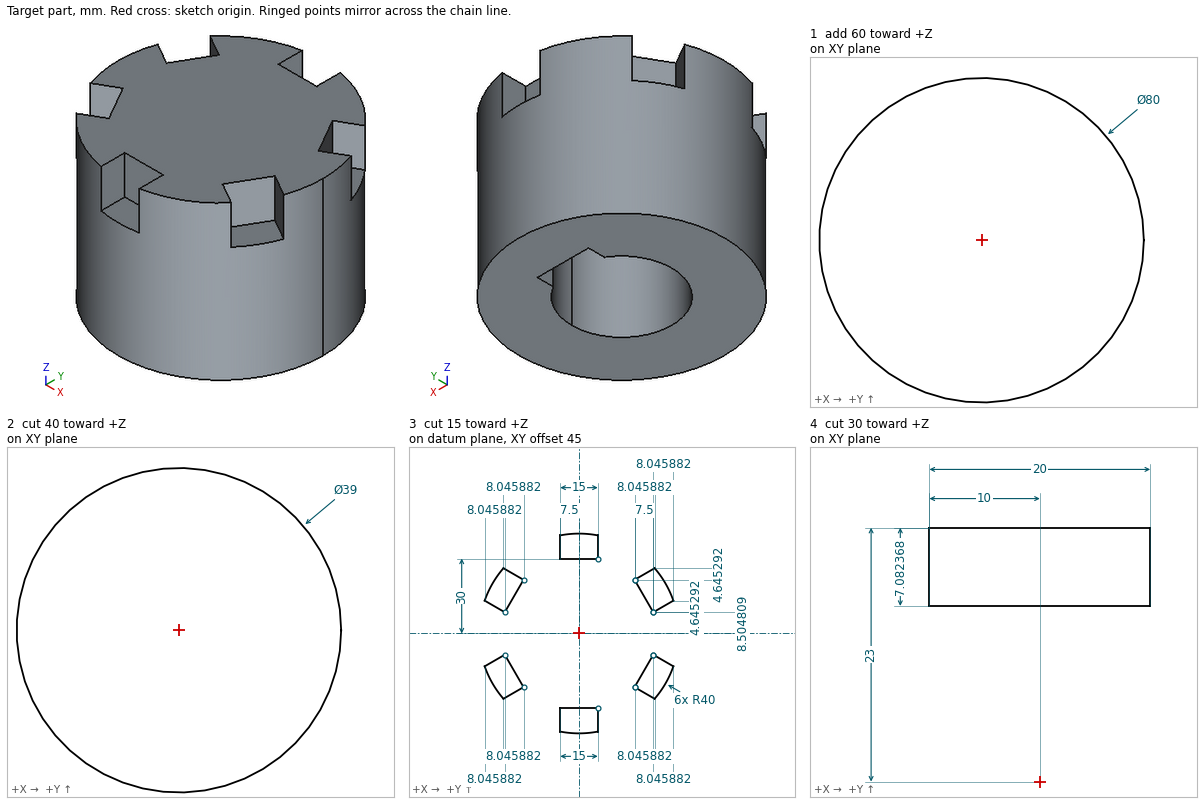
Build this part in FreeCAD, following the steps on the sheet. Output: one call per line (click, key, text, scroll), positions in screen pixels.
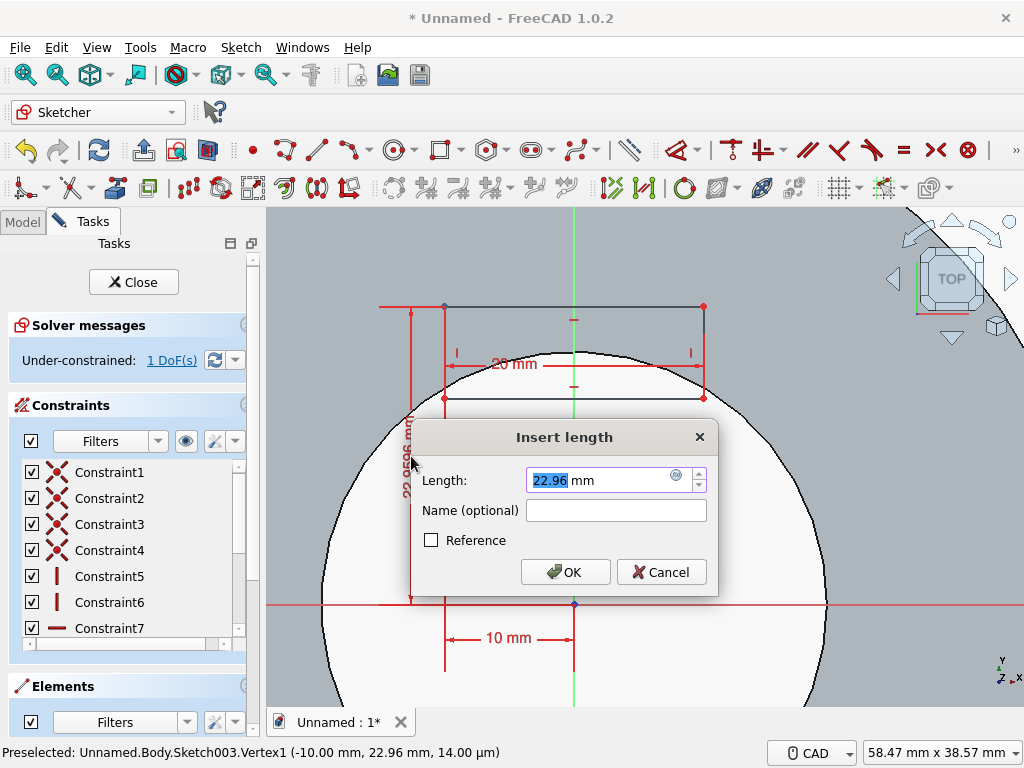
text(23)
key(Return)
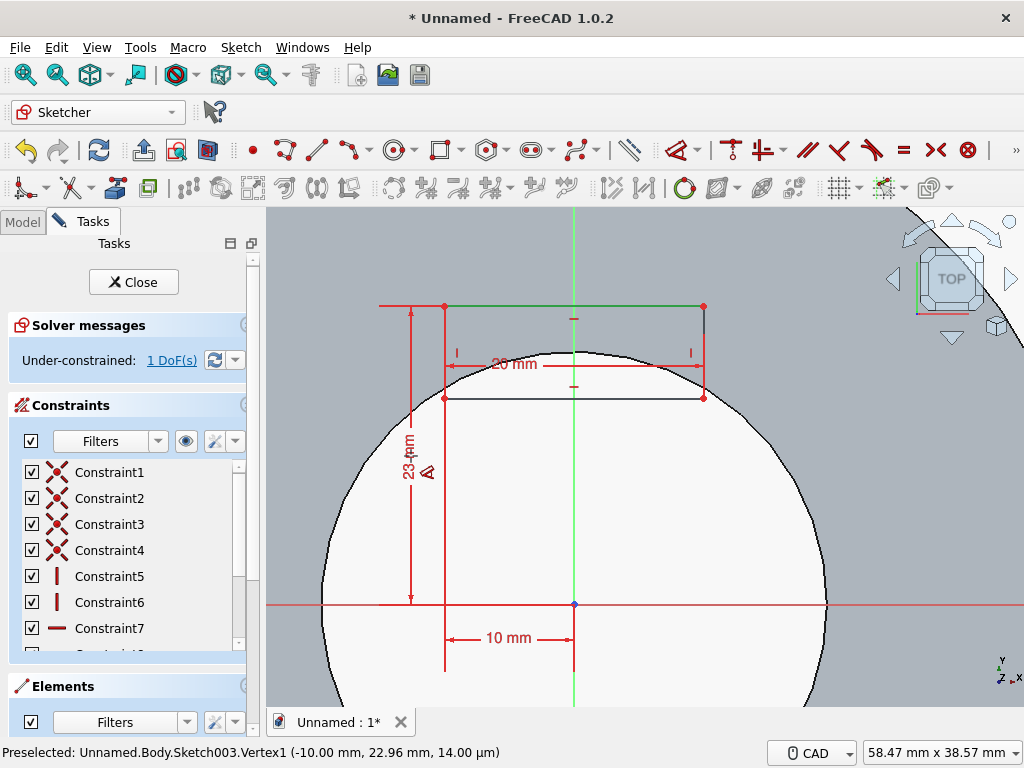
click(445, 334)
click(411, 353)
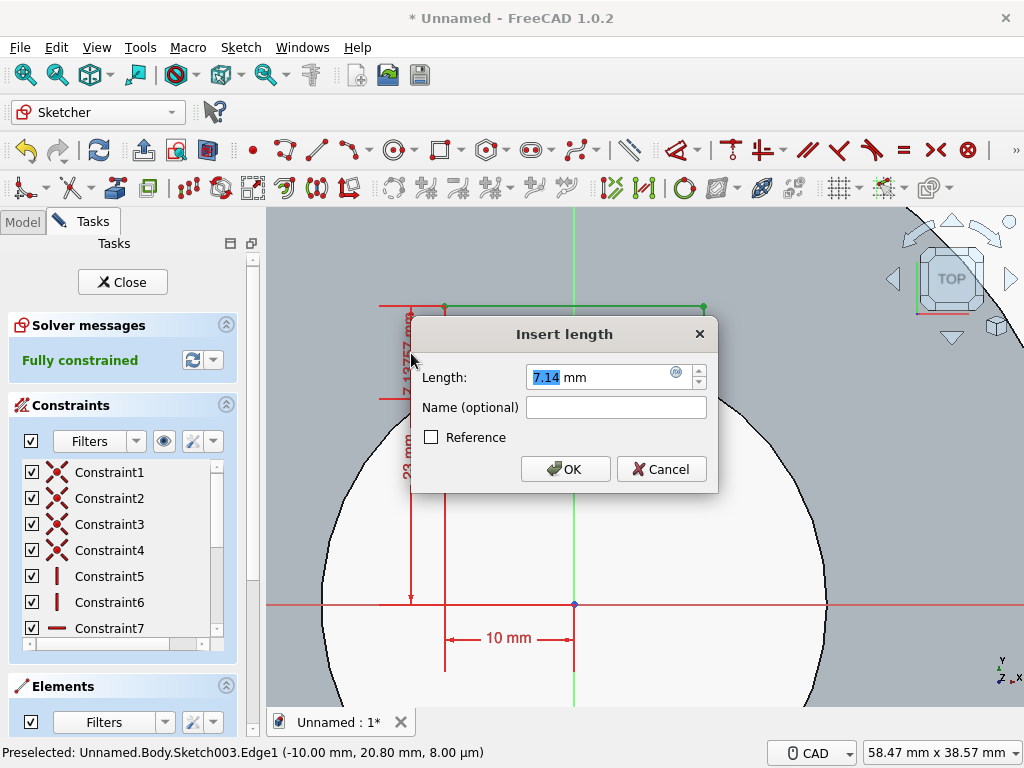
text(7.082368)
key(Return)
key(Escape)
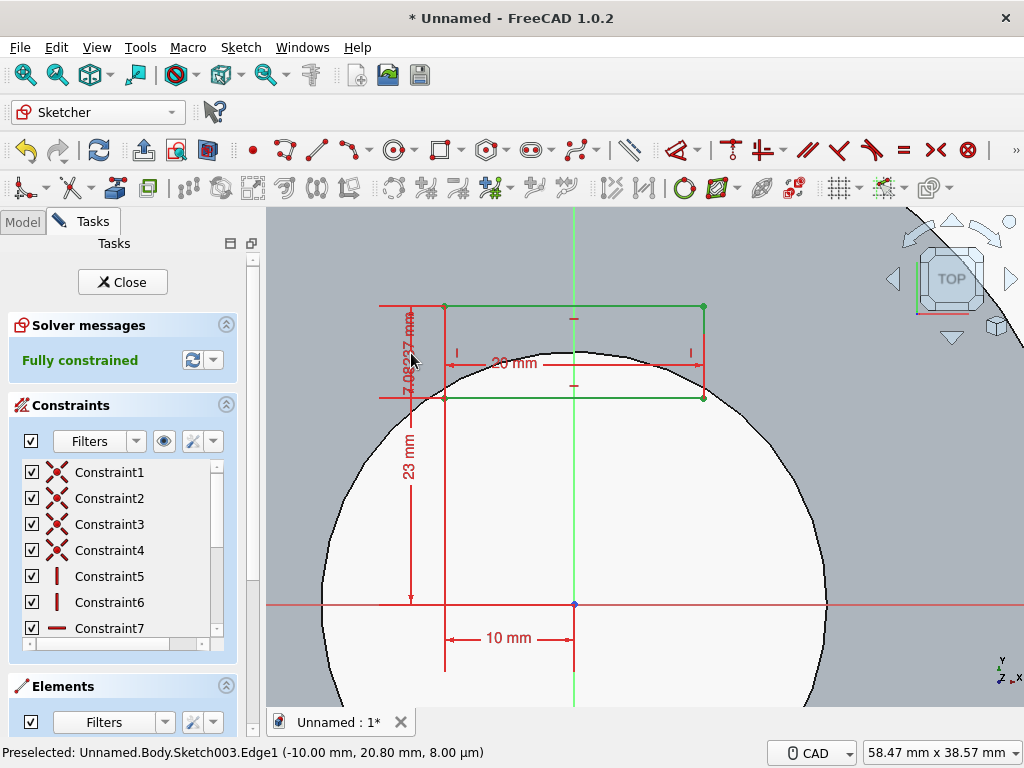
click(123, 282)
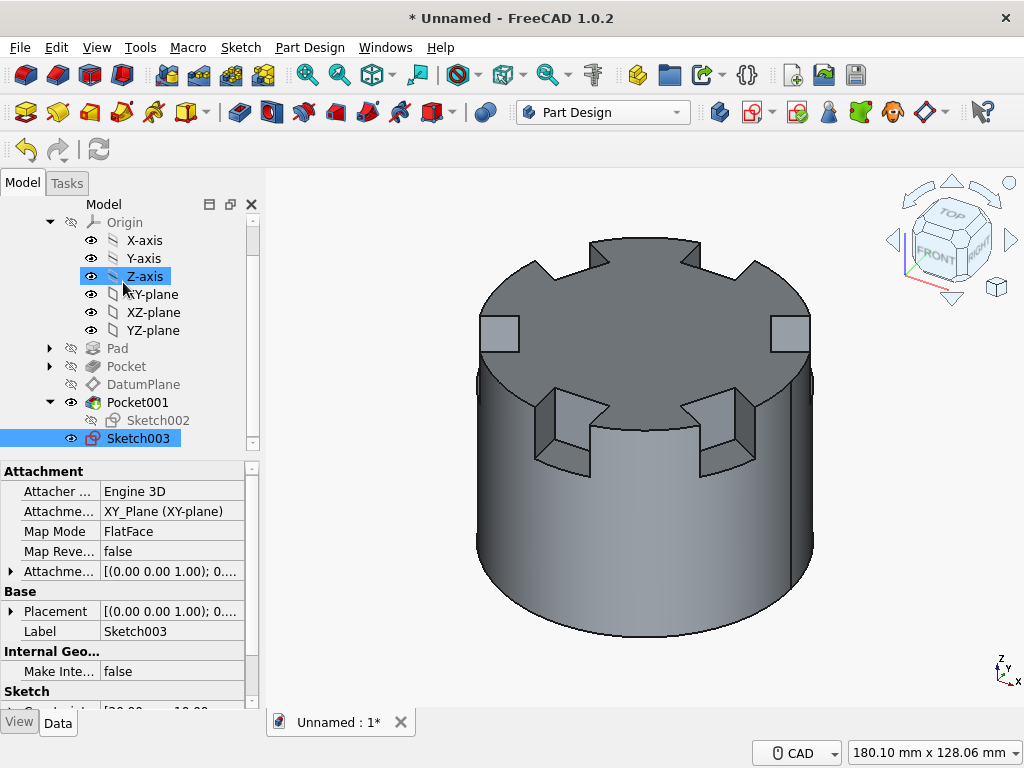
click(240, 112)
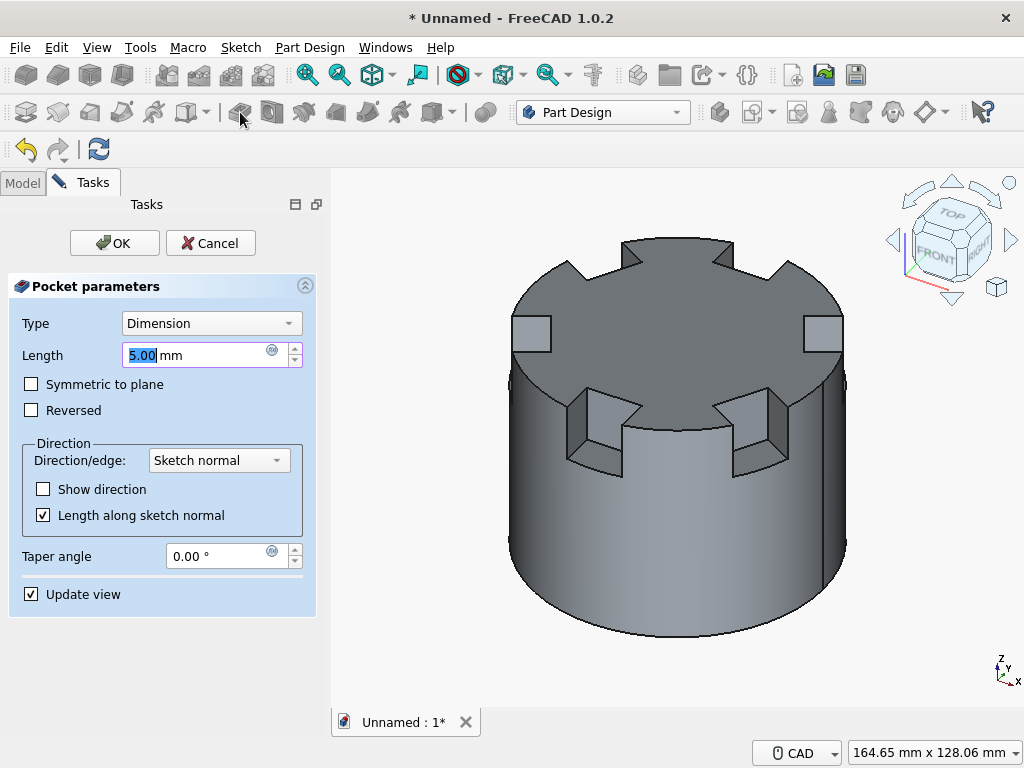
text(30)
key(Tab)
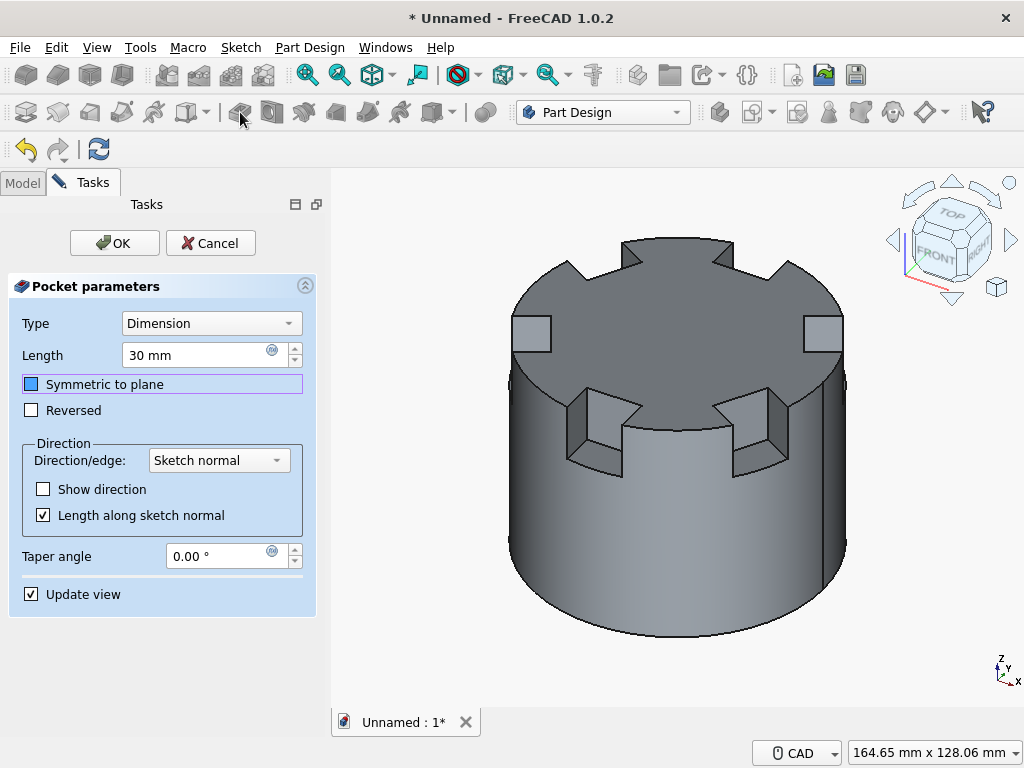
click(30, 410)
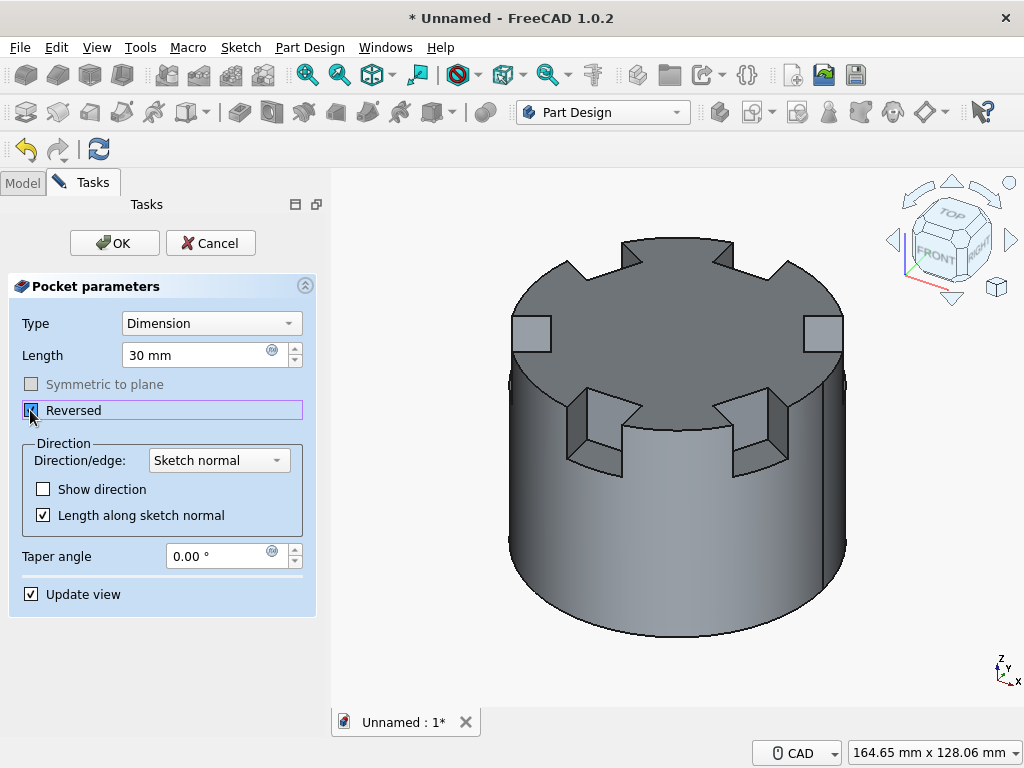
click(115, 243)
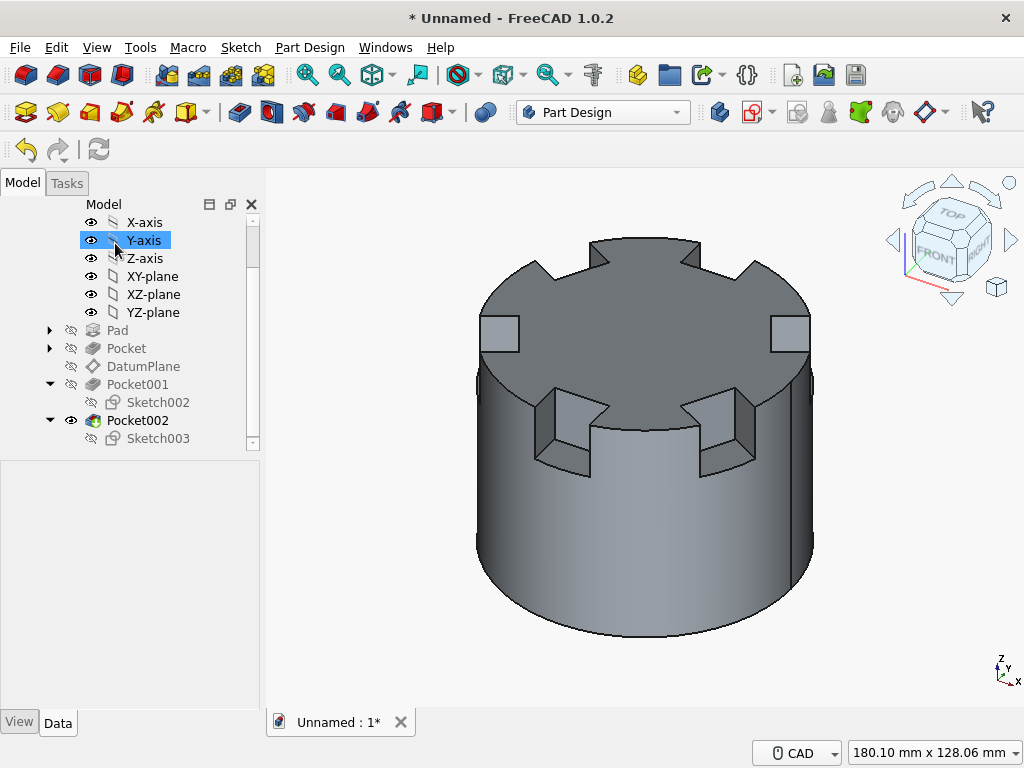
key(0)